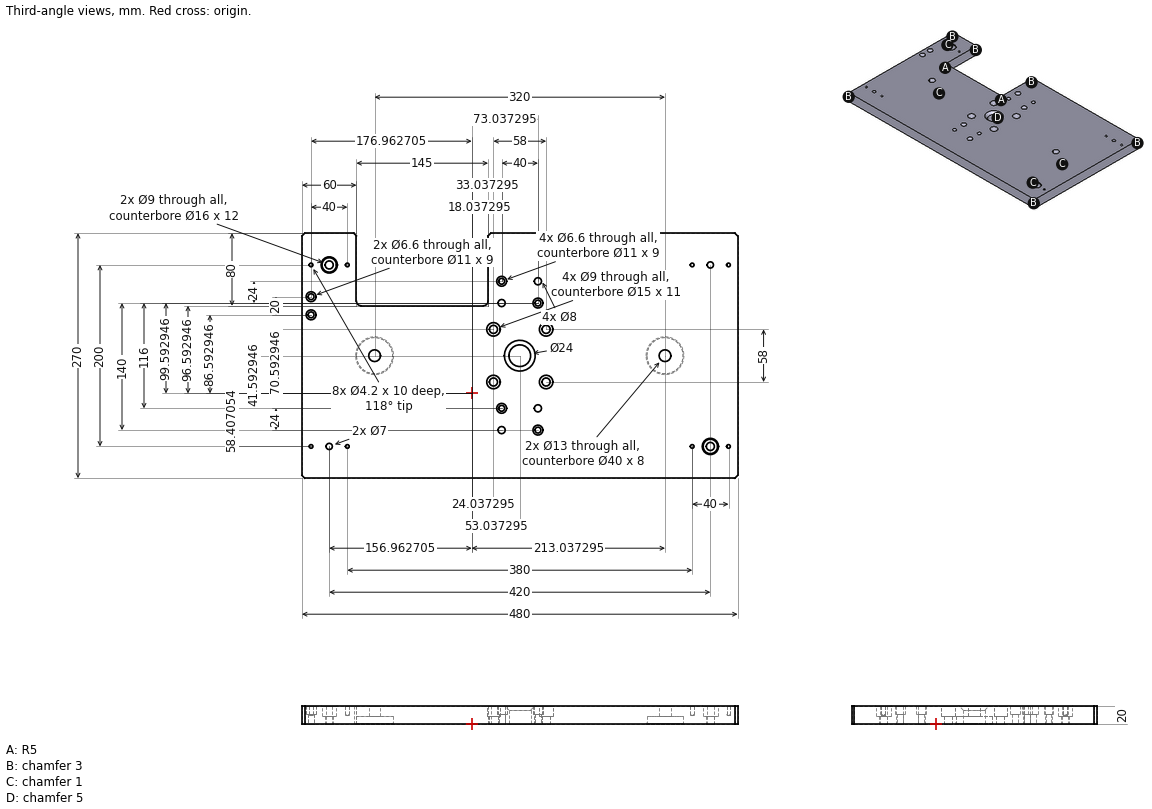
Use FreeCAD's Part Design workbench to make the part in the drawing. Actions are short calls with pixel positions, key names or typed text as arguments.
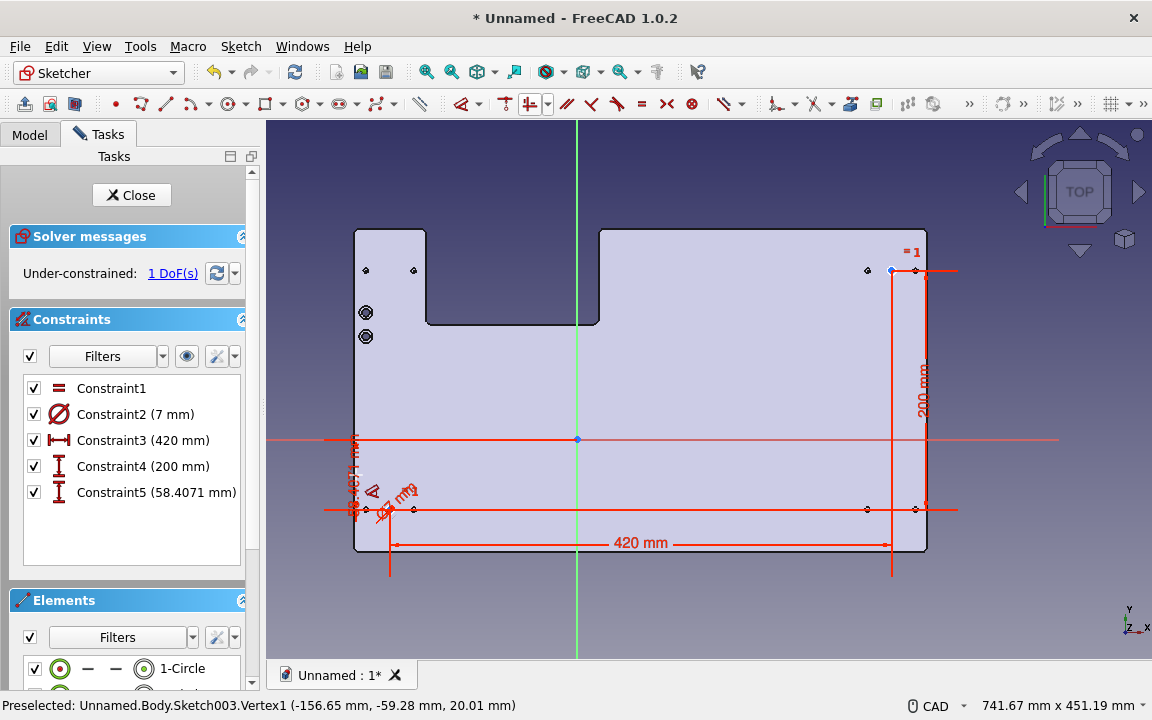
click(390, 510)
click(484, 544)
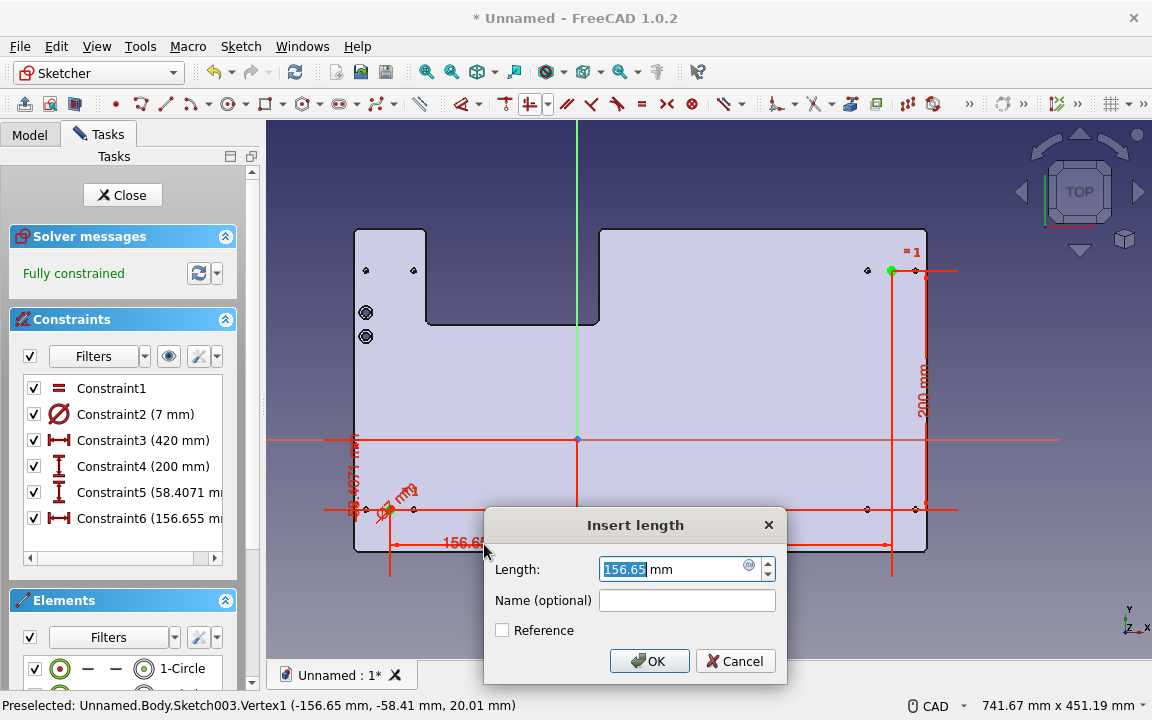
text(156.962705)
key(Return)
key(Escape)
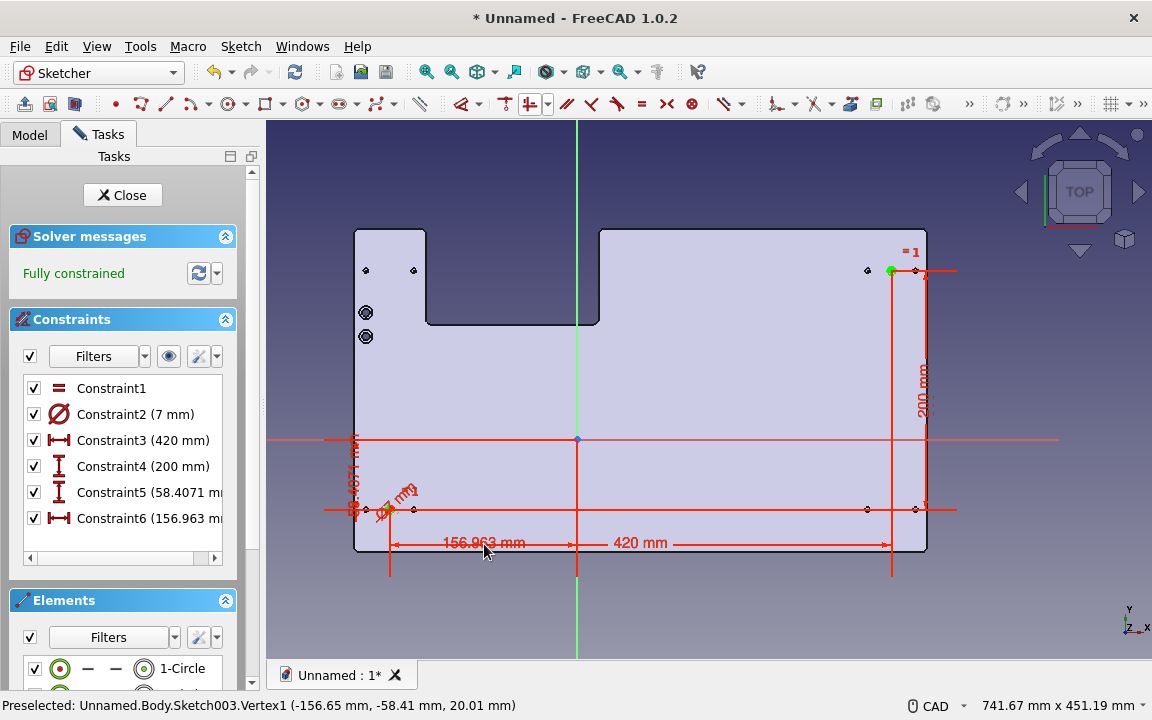
click(123, 195)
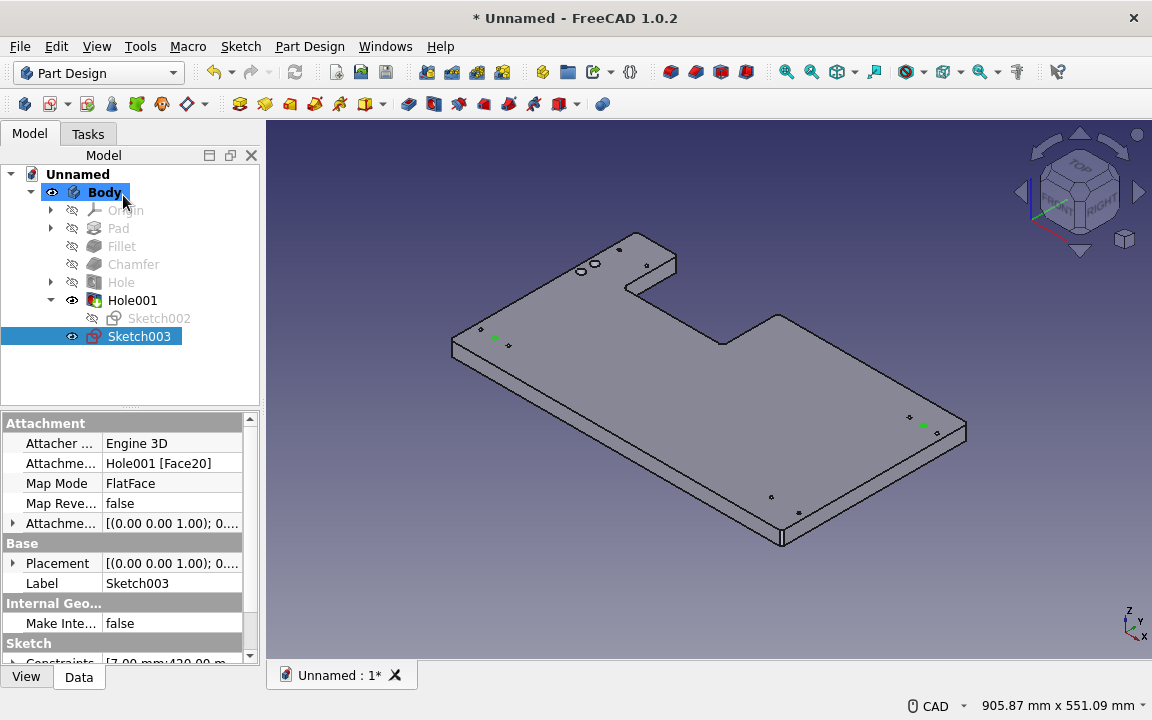
click(409, 104)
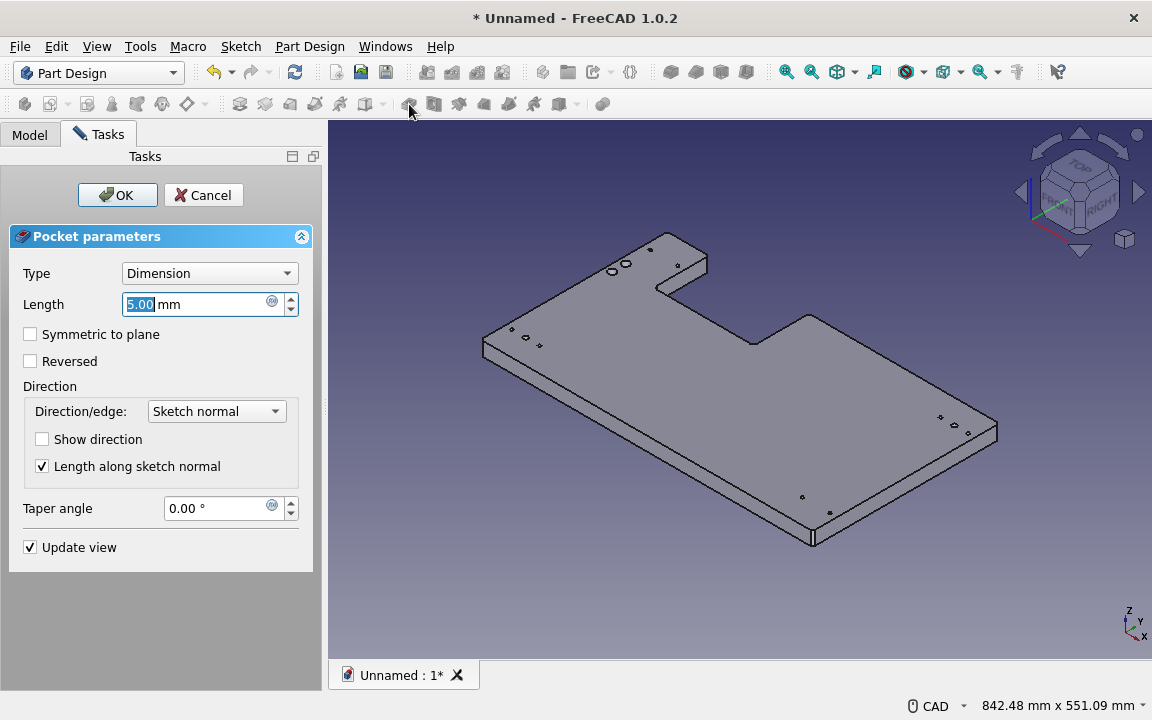
click(210, 274)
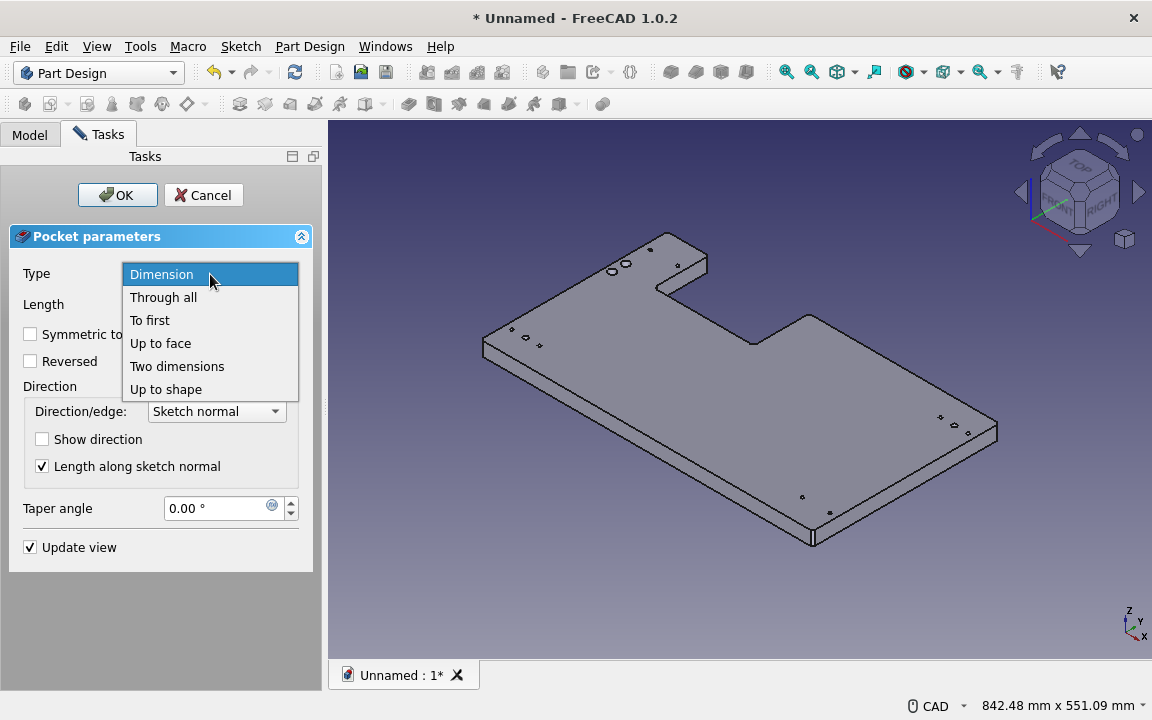
click(208, 298)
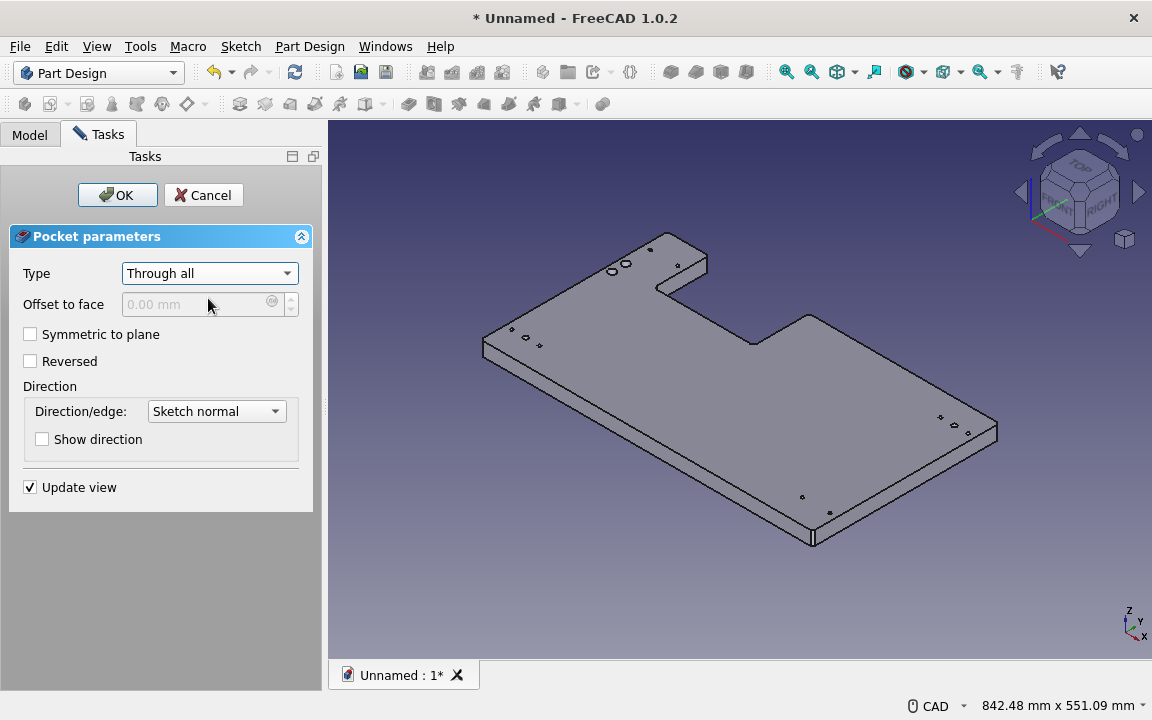
click(118, 195)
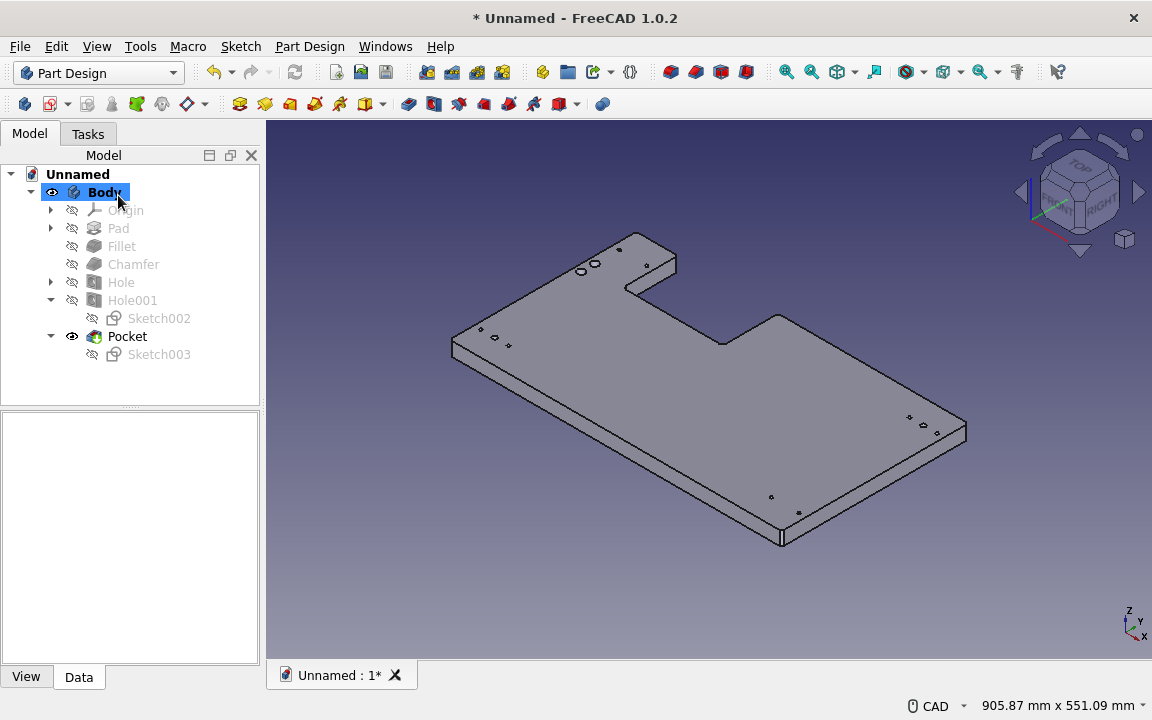
click(756, 408)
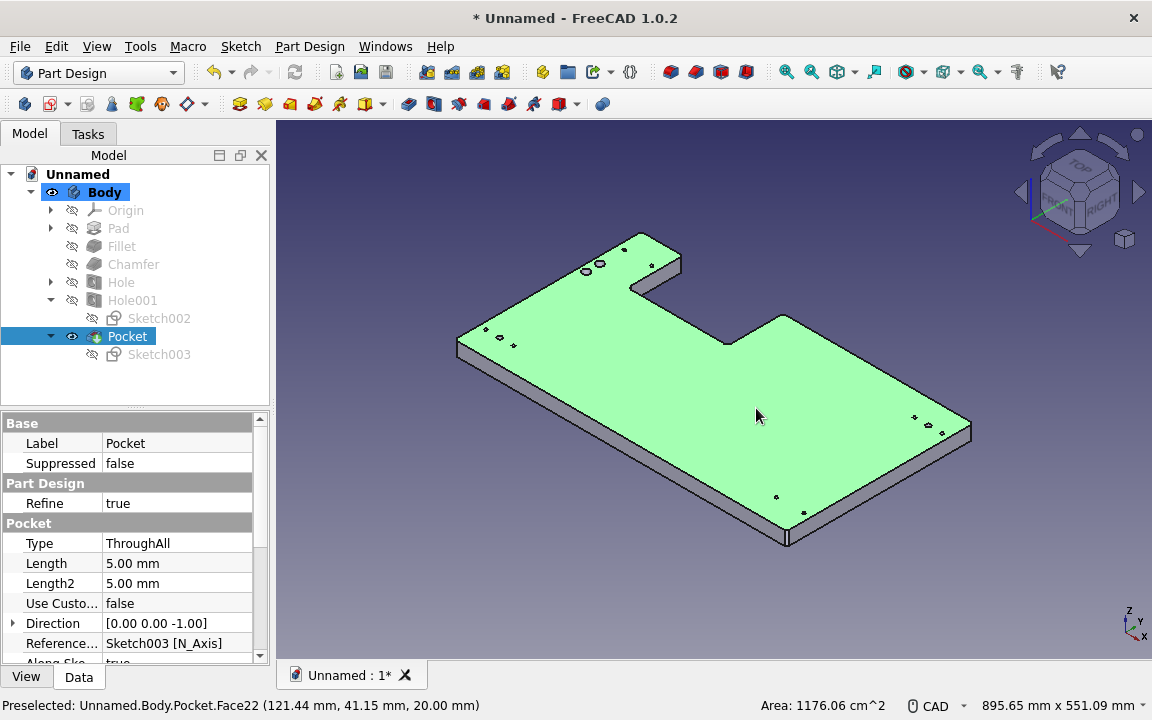
click(50, 104)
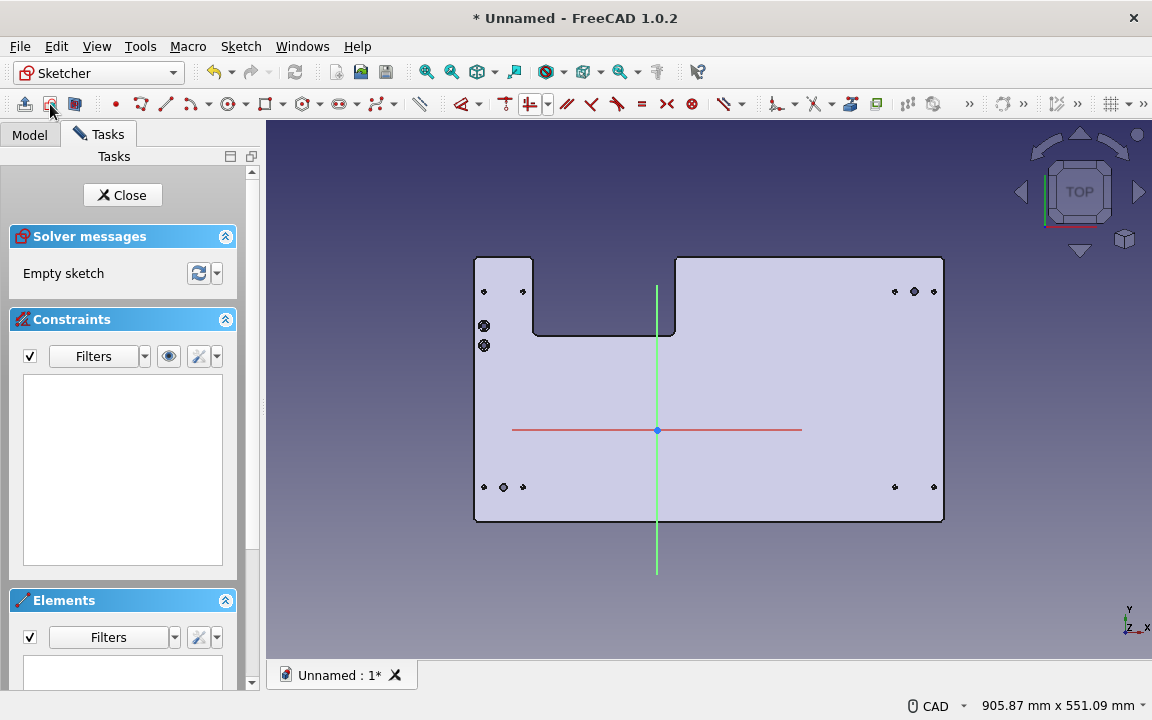
click(228, 104)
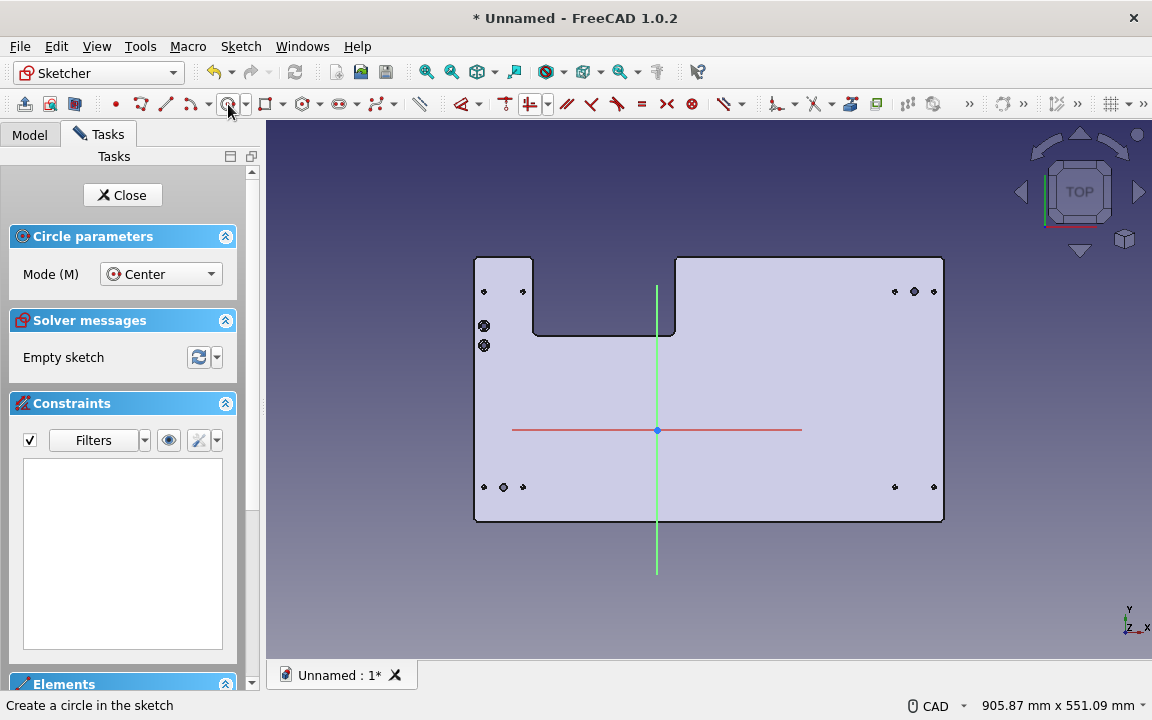
scroll(504, 292, up, 9)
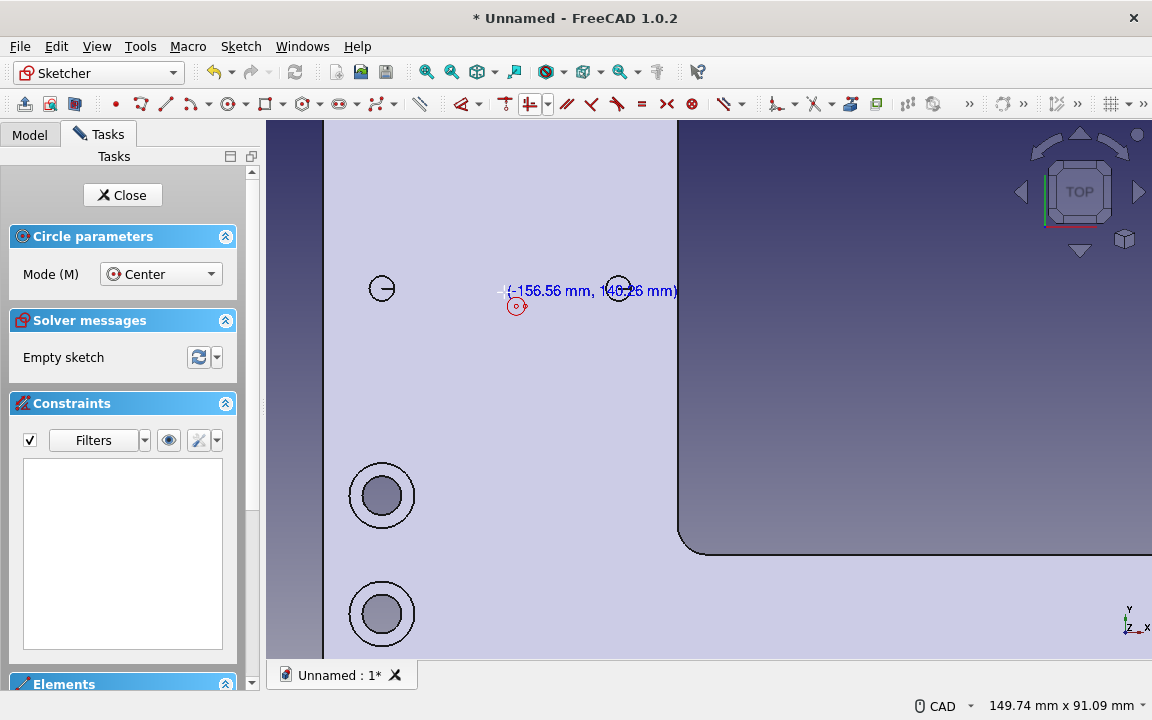
scroll(362, 265, down, 8)